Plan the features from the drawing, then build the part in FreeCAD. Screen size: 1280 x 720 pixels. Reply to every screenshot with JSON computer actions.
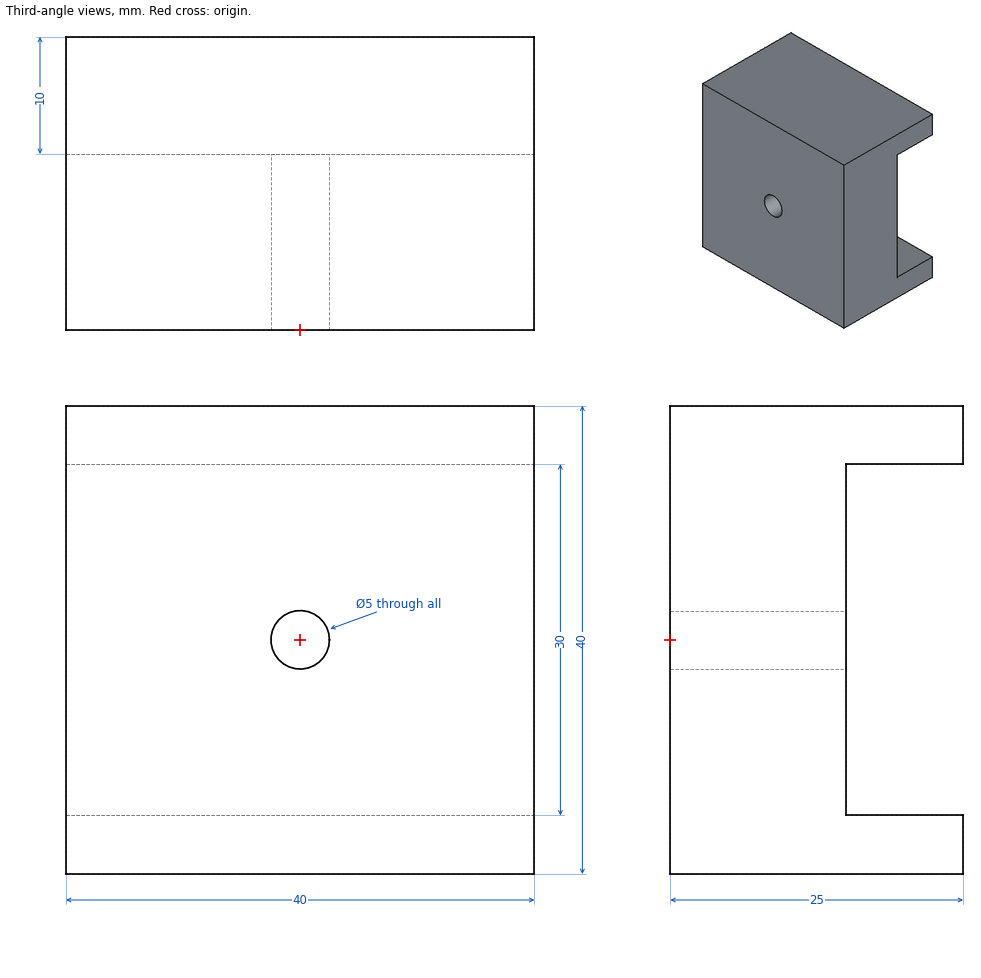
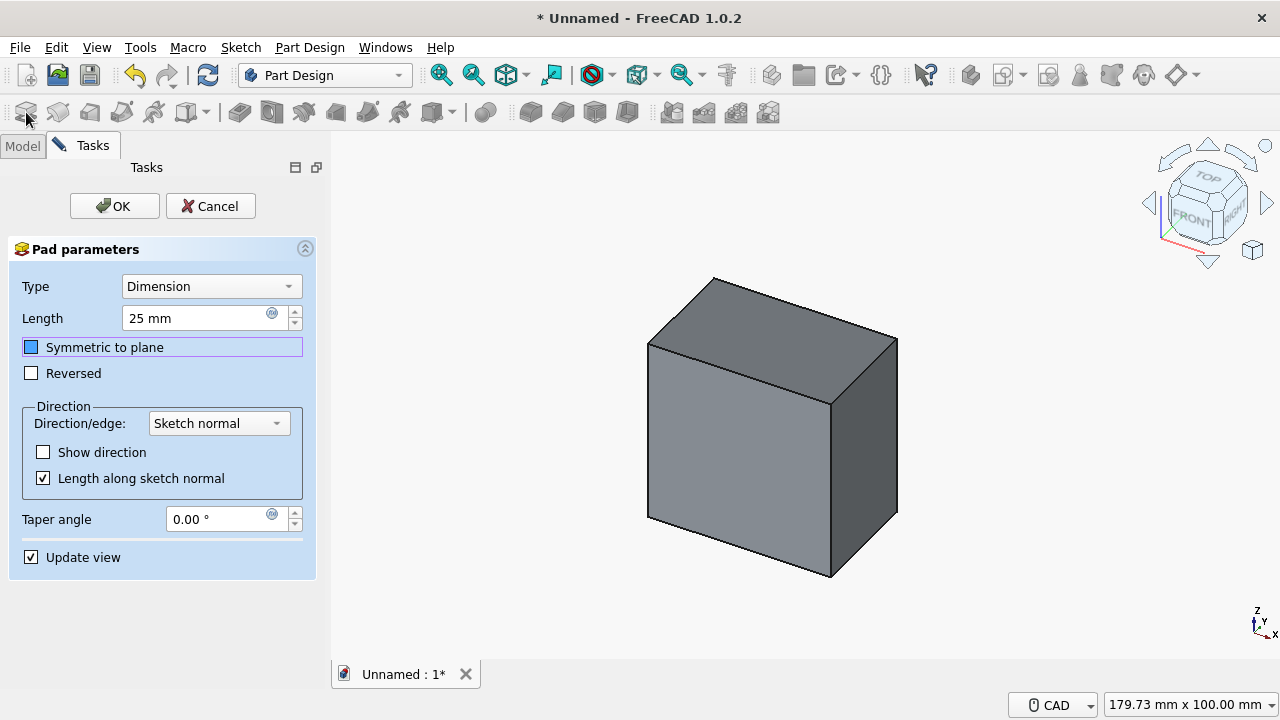
{"action": "left_click", "coordinate": [30, 373]}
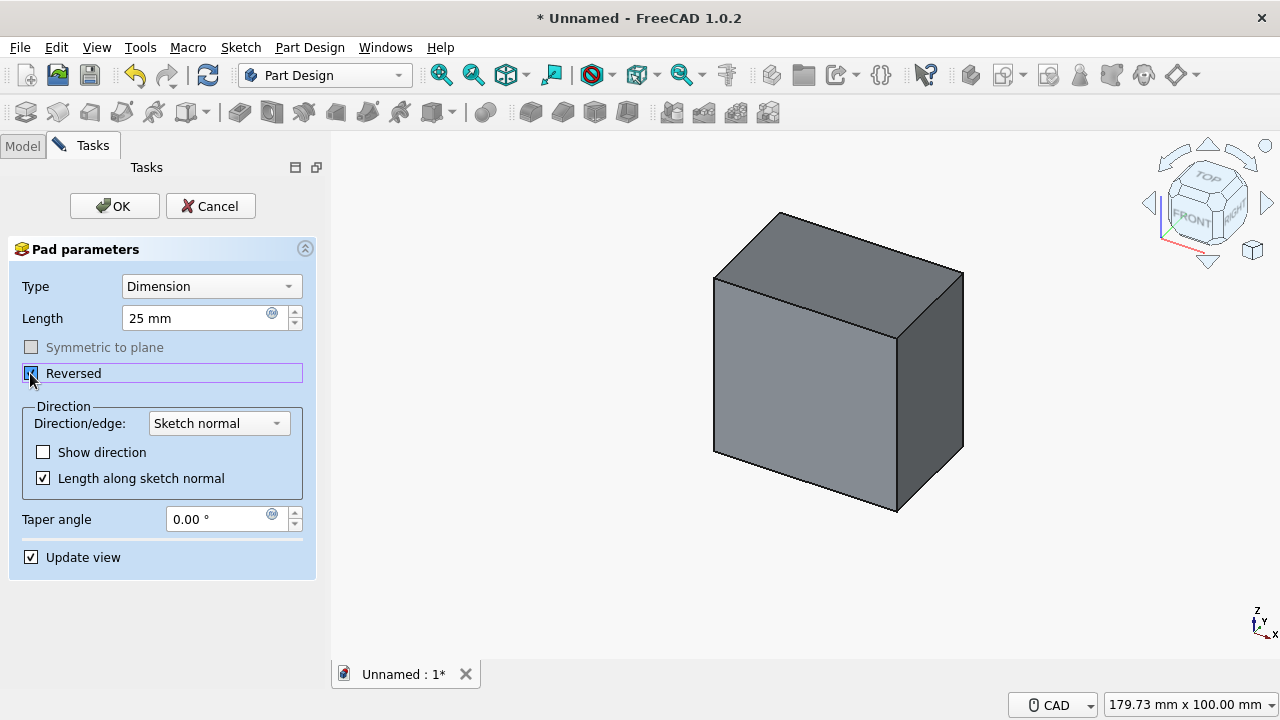
{"action": "left_click", "coordinate": [115, 206]}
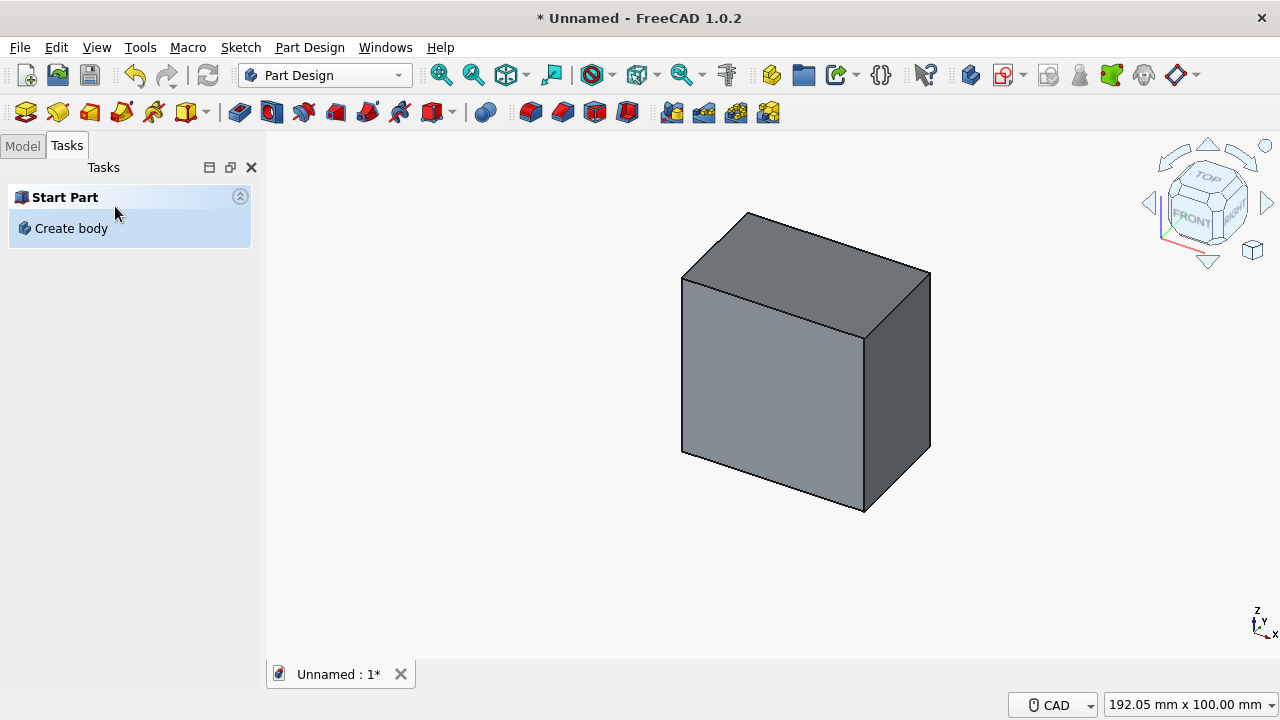
{"action": "key", "text": "4"}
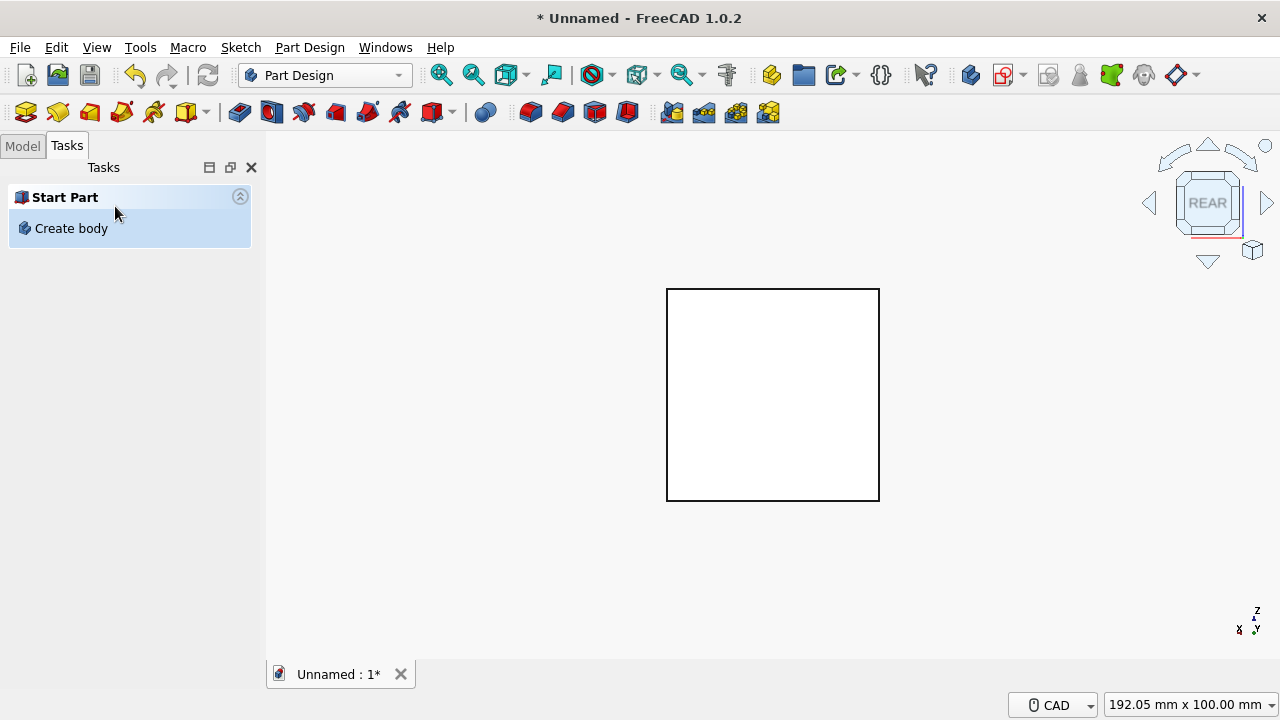
{"action": "left_click", "coordinate": [442, 76]}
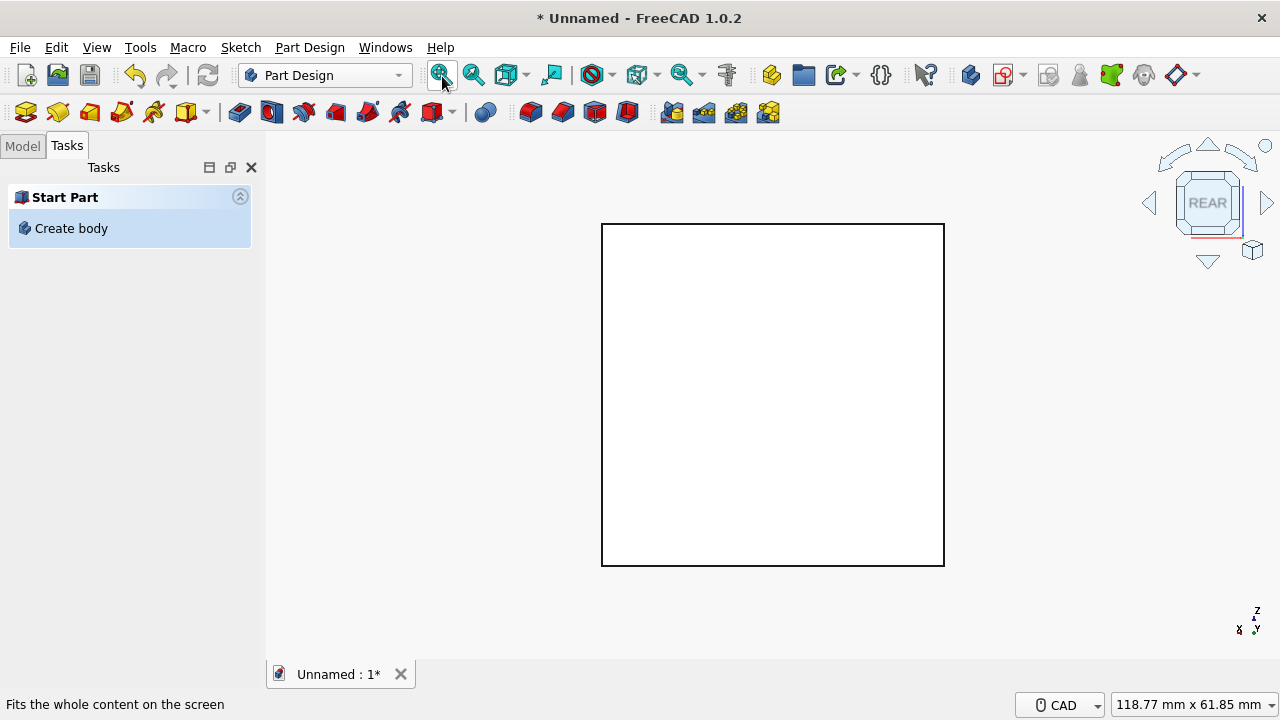
{"action": "left_click", "coordinate": [773, 394]}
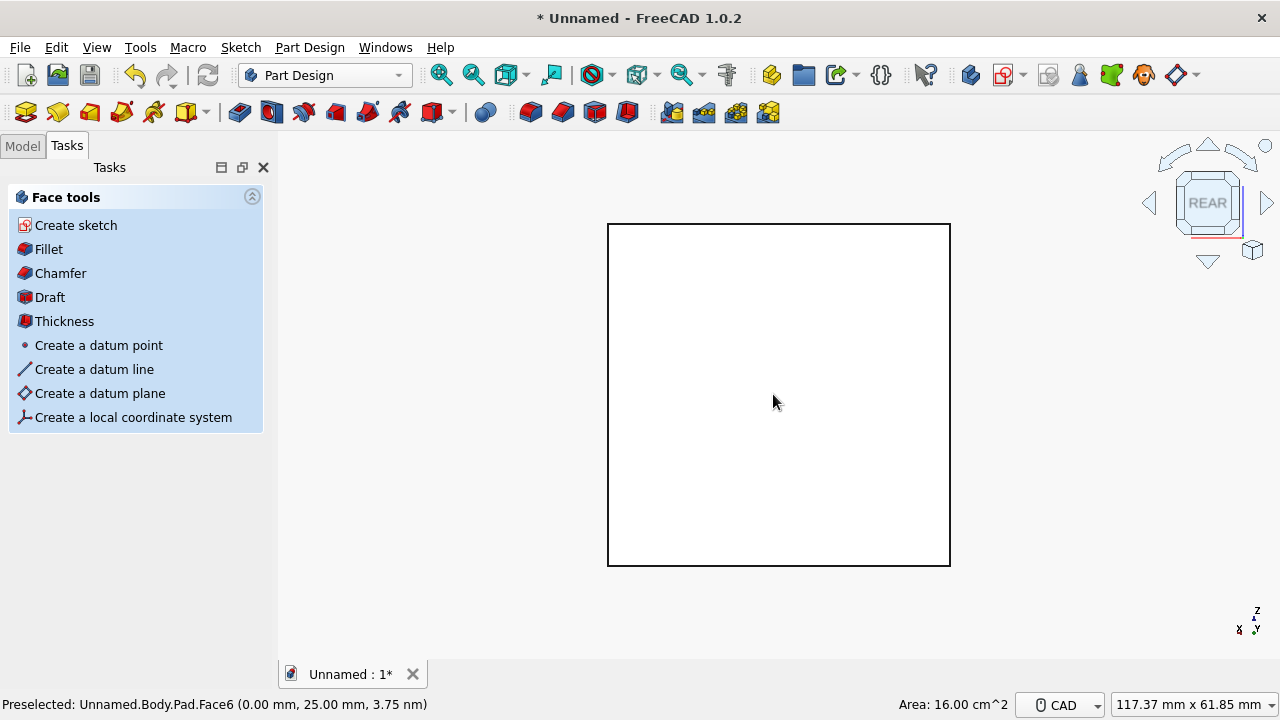
{"action": "left_click", "coordinate": [1004, 76]}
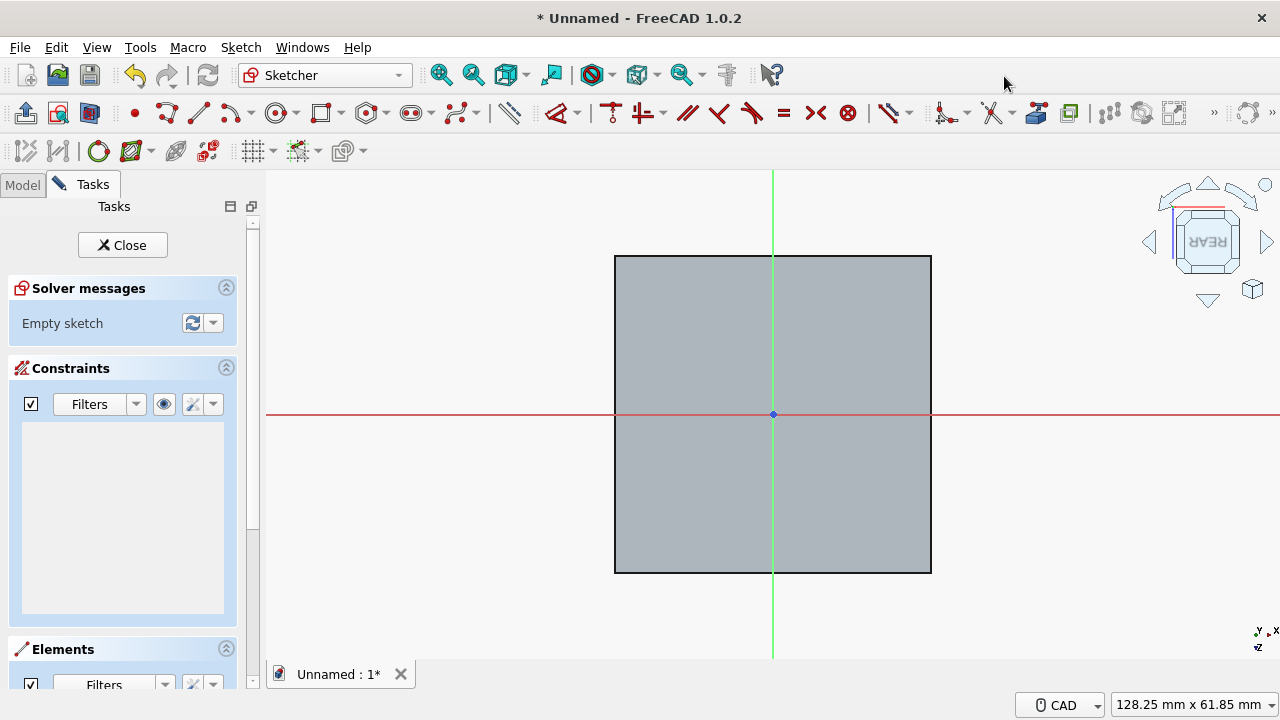
{"action": "left_click", "coordinate": [344, 114]}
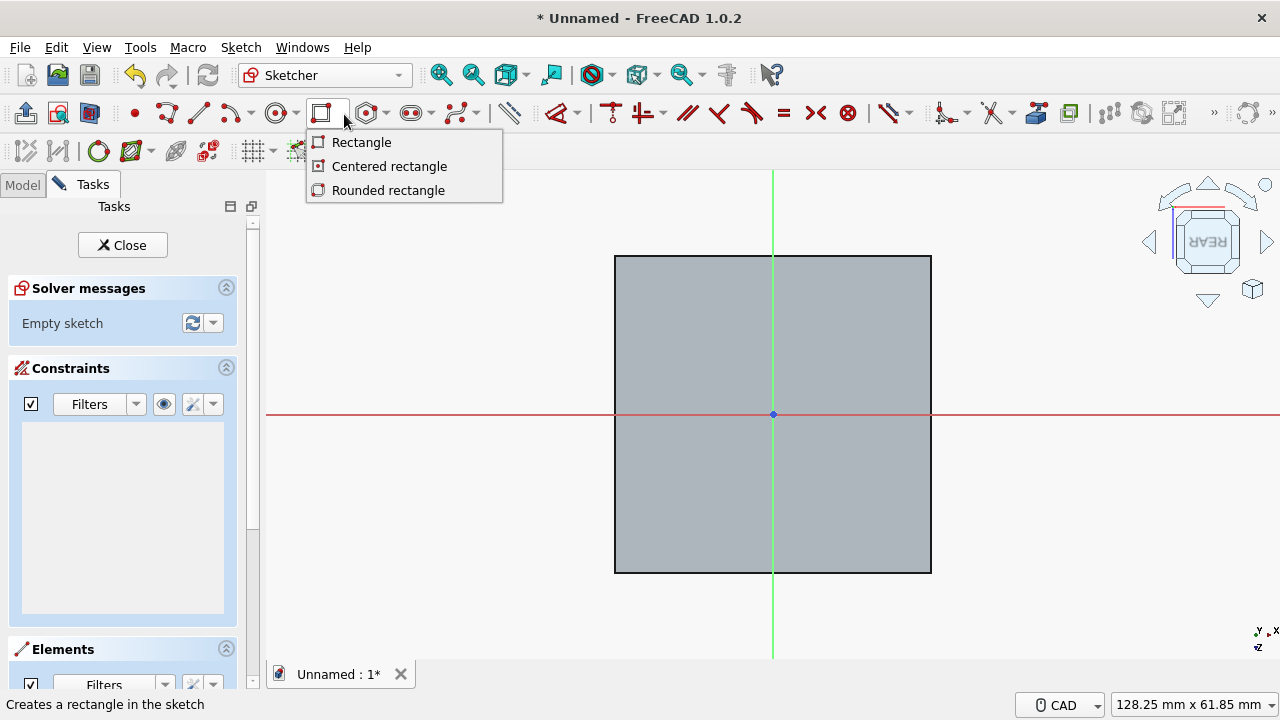
{"action": "left_click", "coordinate": [404, 166]}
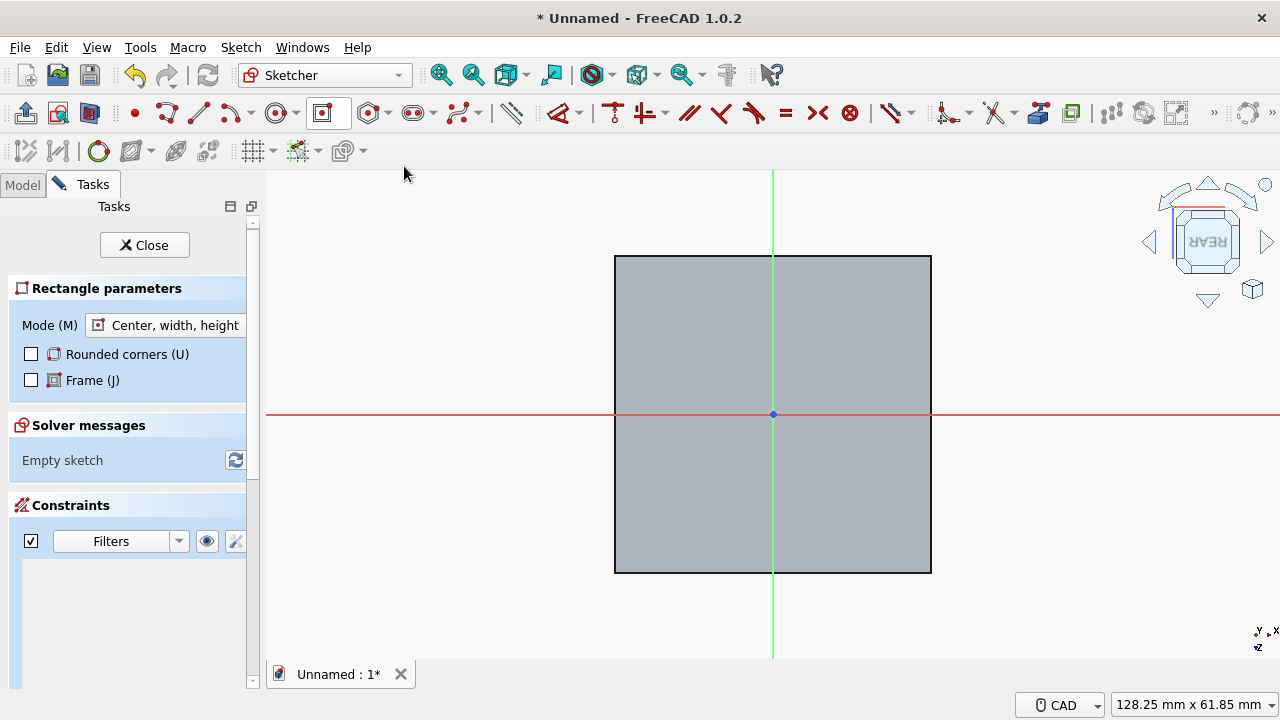
{"action": "left_click", "coordinate": [773, 414]}
{"action": "mouse_move", "coordinate": [931, 296]}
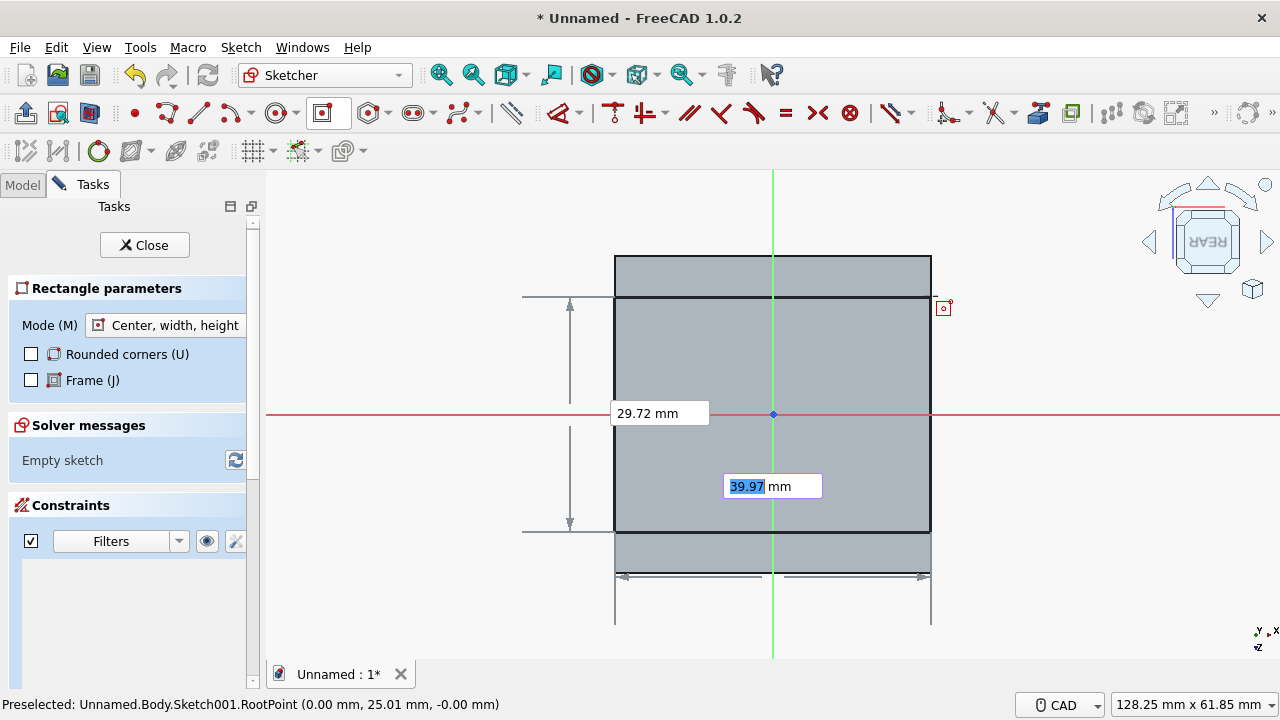
{"action": "type", "text": "40"}
{"action": "key", "text": "Tab"}
{"action": "type", "text": "30"}
{"action": "key", "text": "Return"}
{"action": "key", "text": "Escape"}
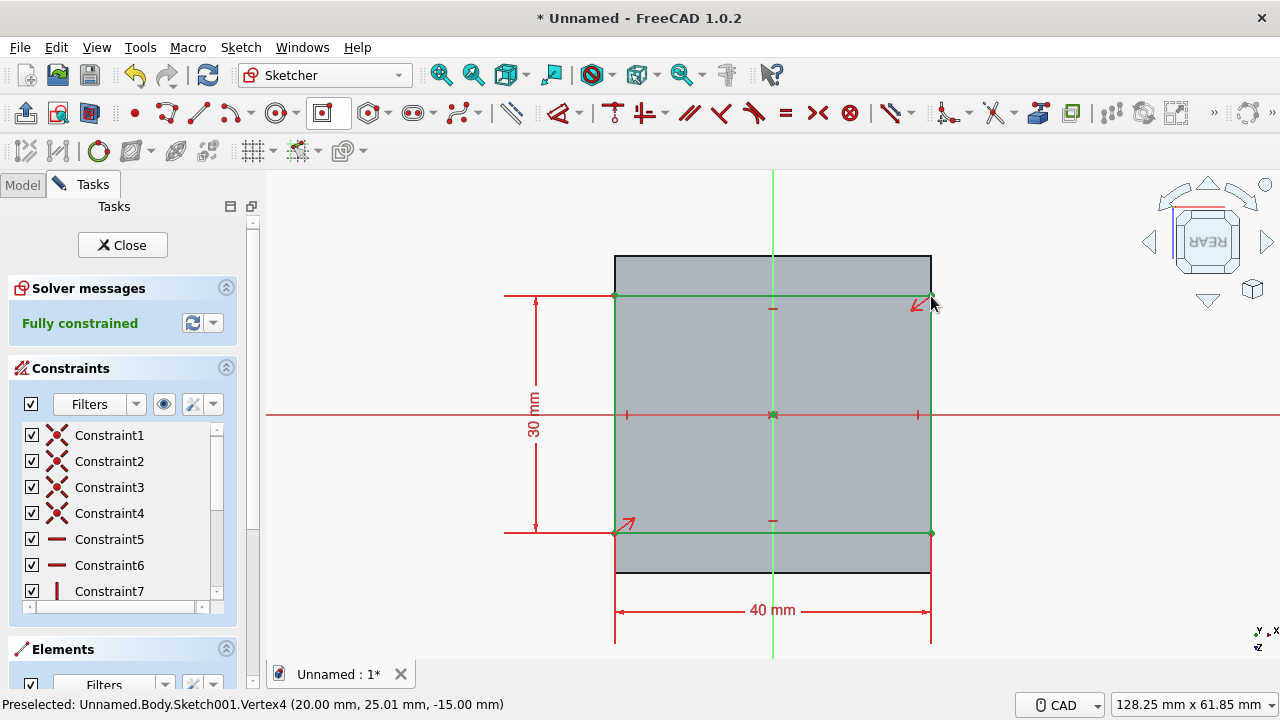
{"action": "left_click", "coordinate": [123, 245]}